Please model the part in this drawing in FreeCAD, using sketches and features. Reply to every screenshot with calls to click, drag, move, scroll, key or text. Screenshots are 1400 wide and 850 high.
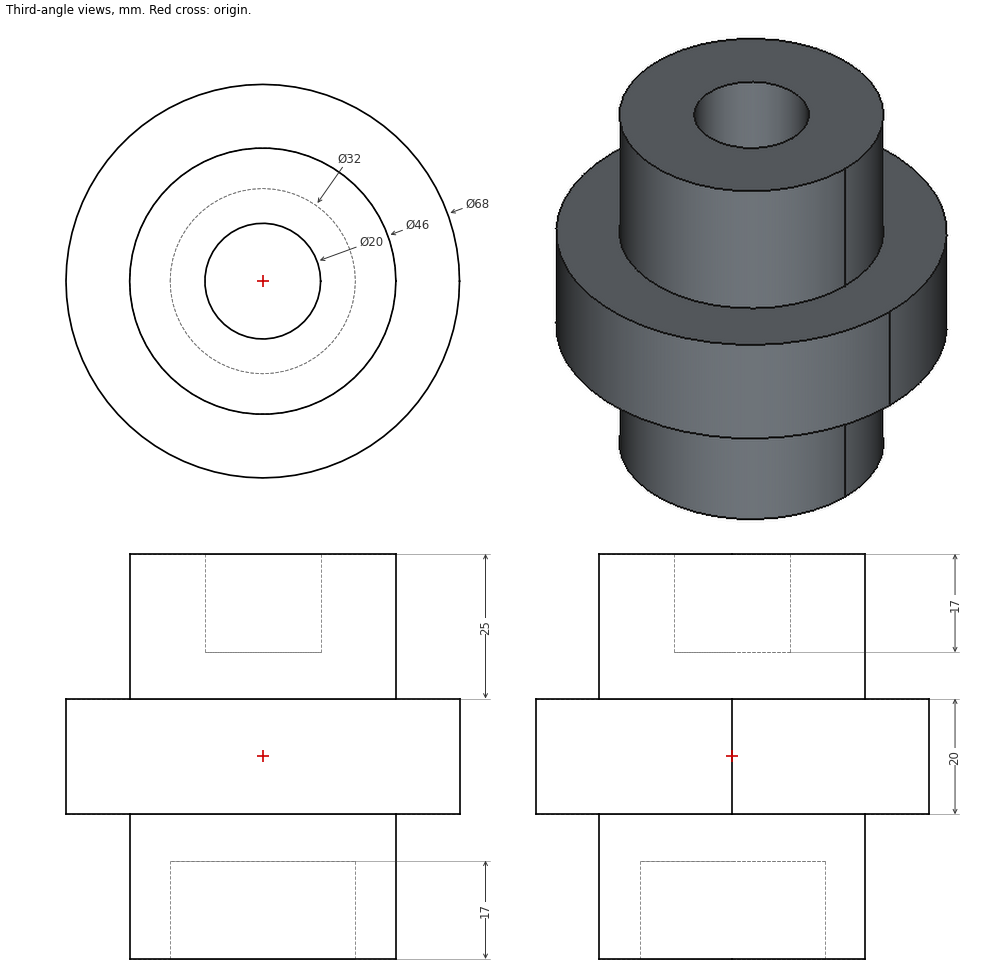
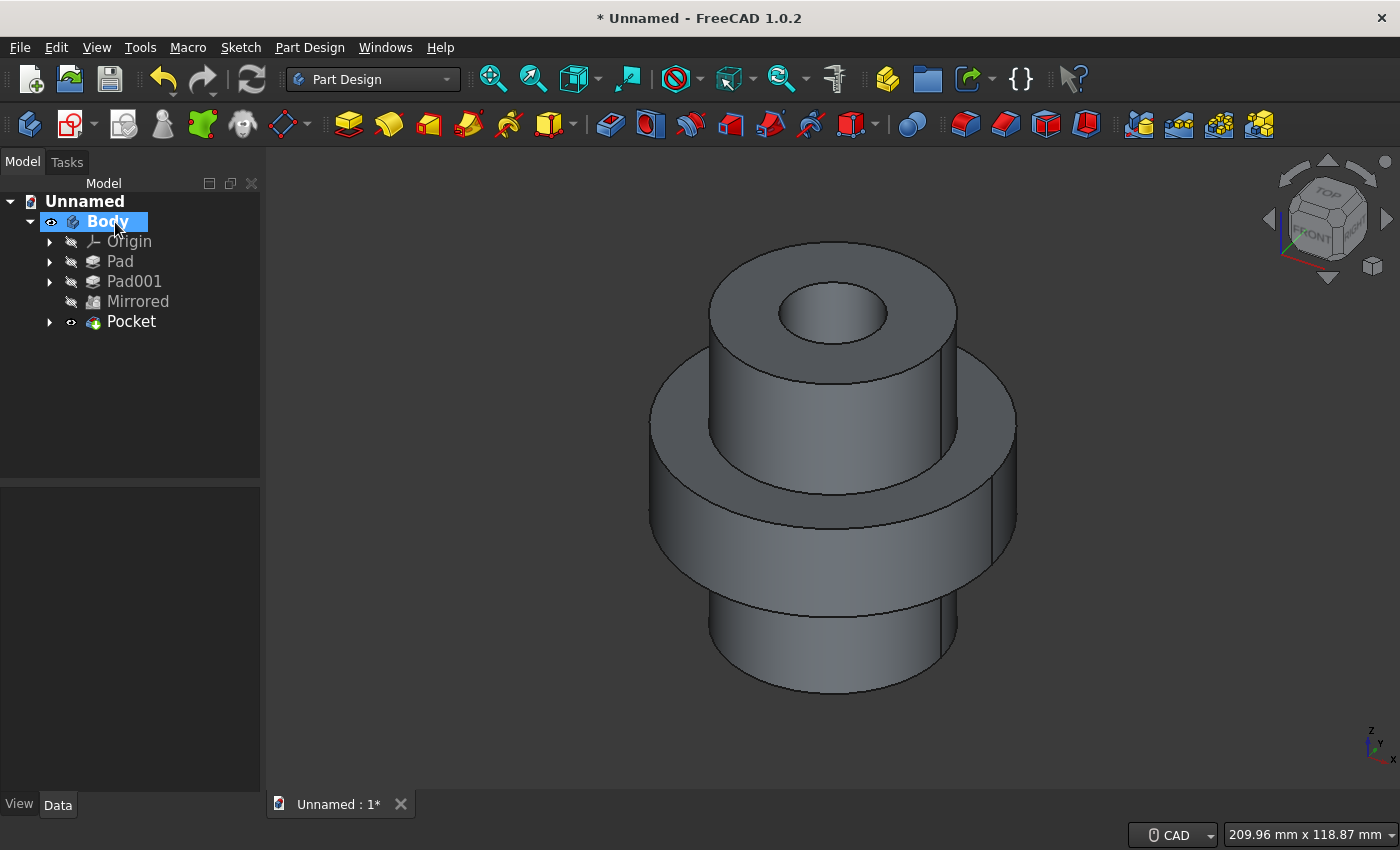
key(5)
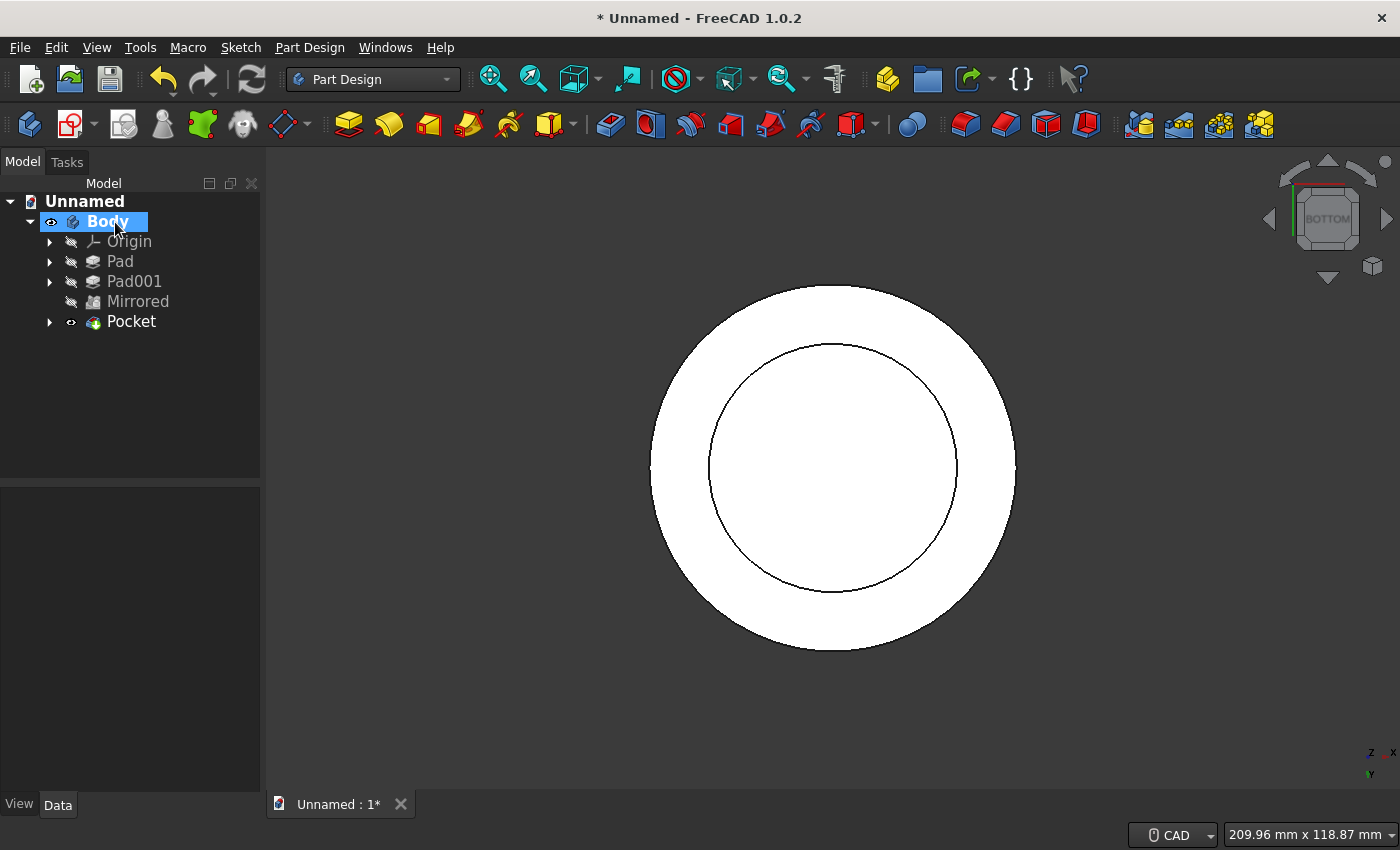
click(833, 467)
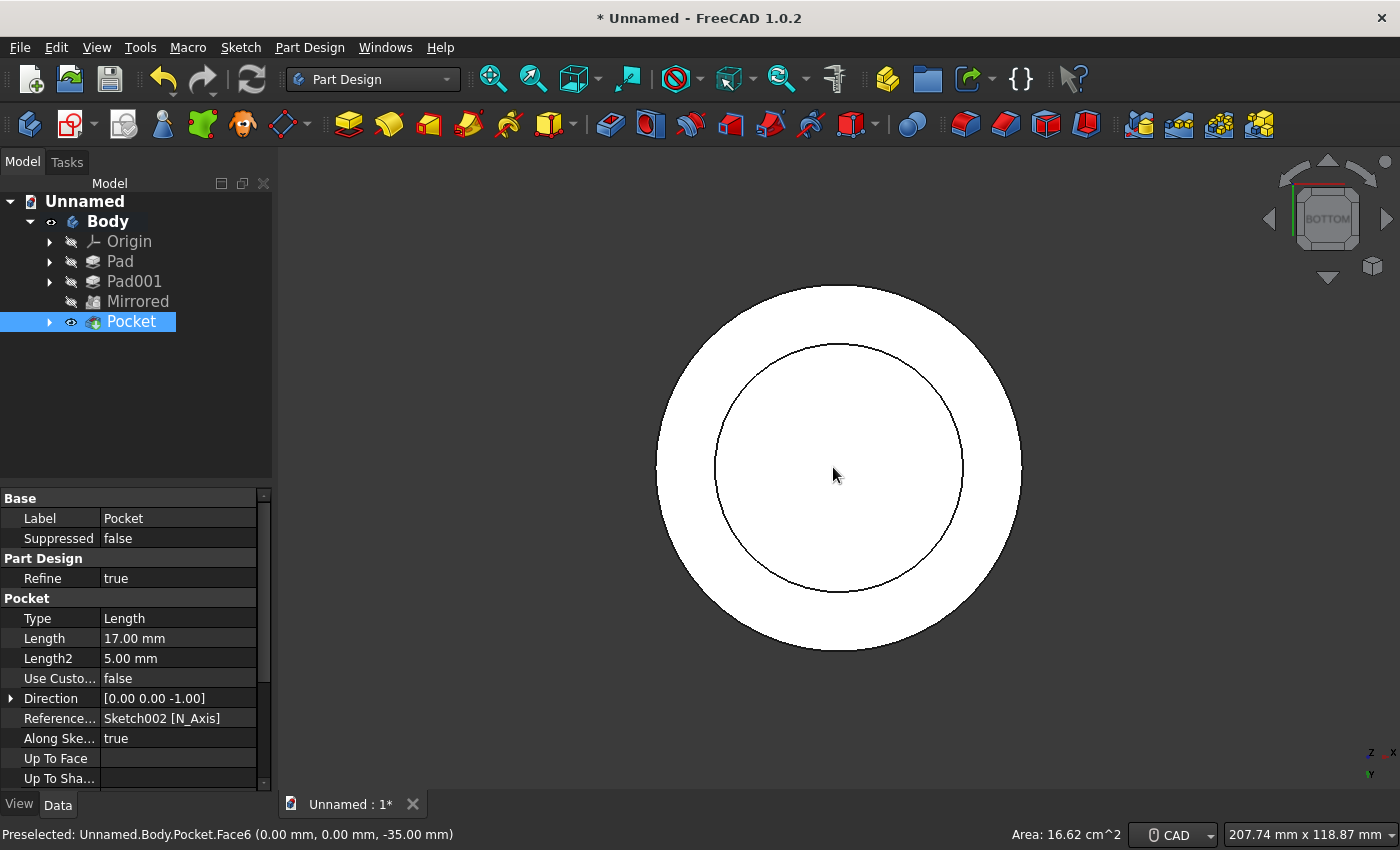
click(70, 124)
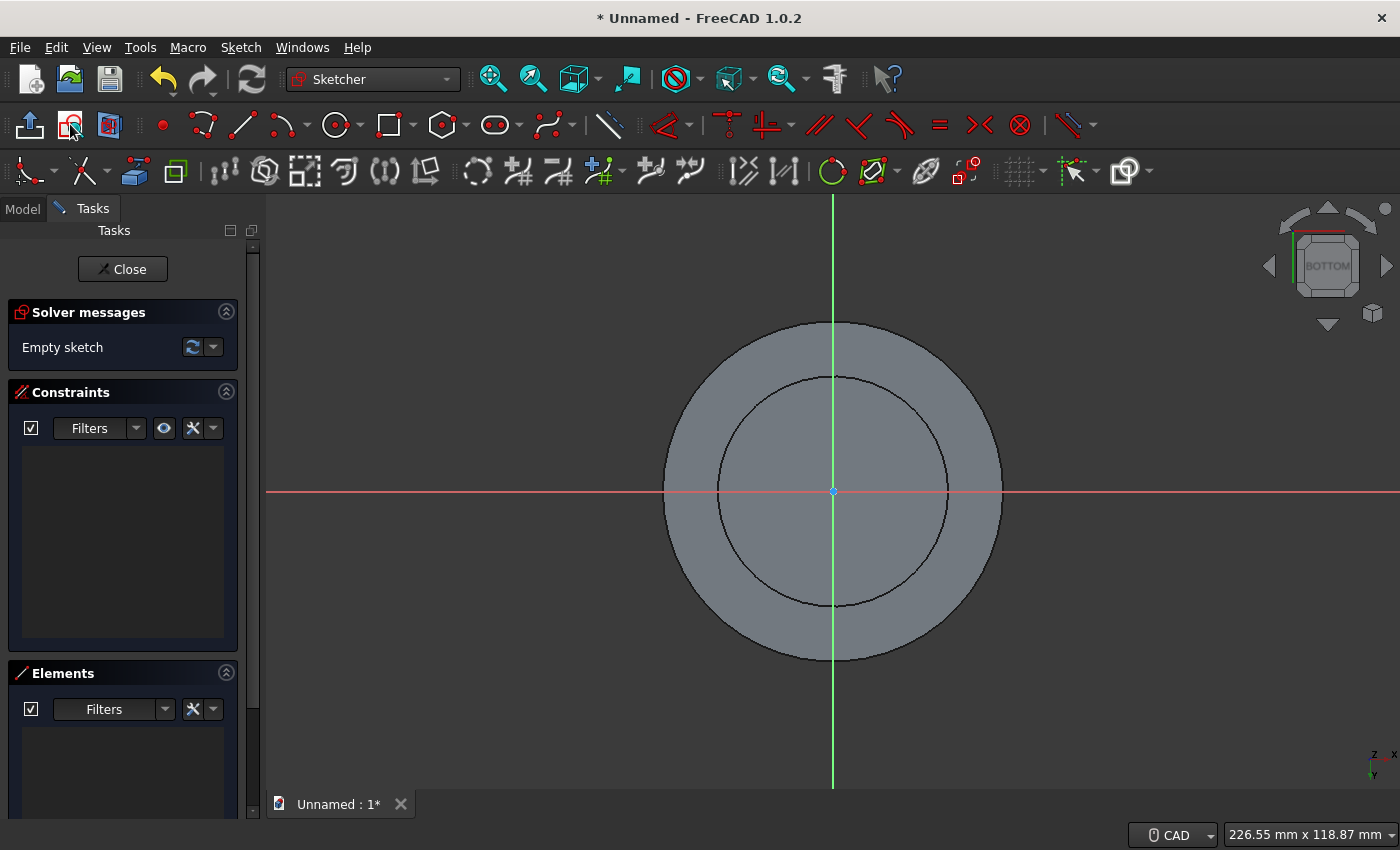
scroll(889, 491, up, 4)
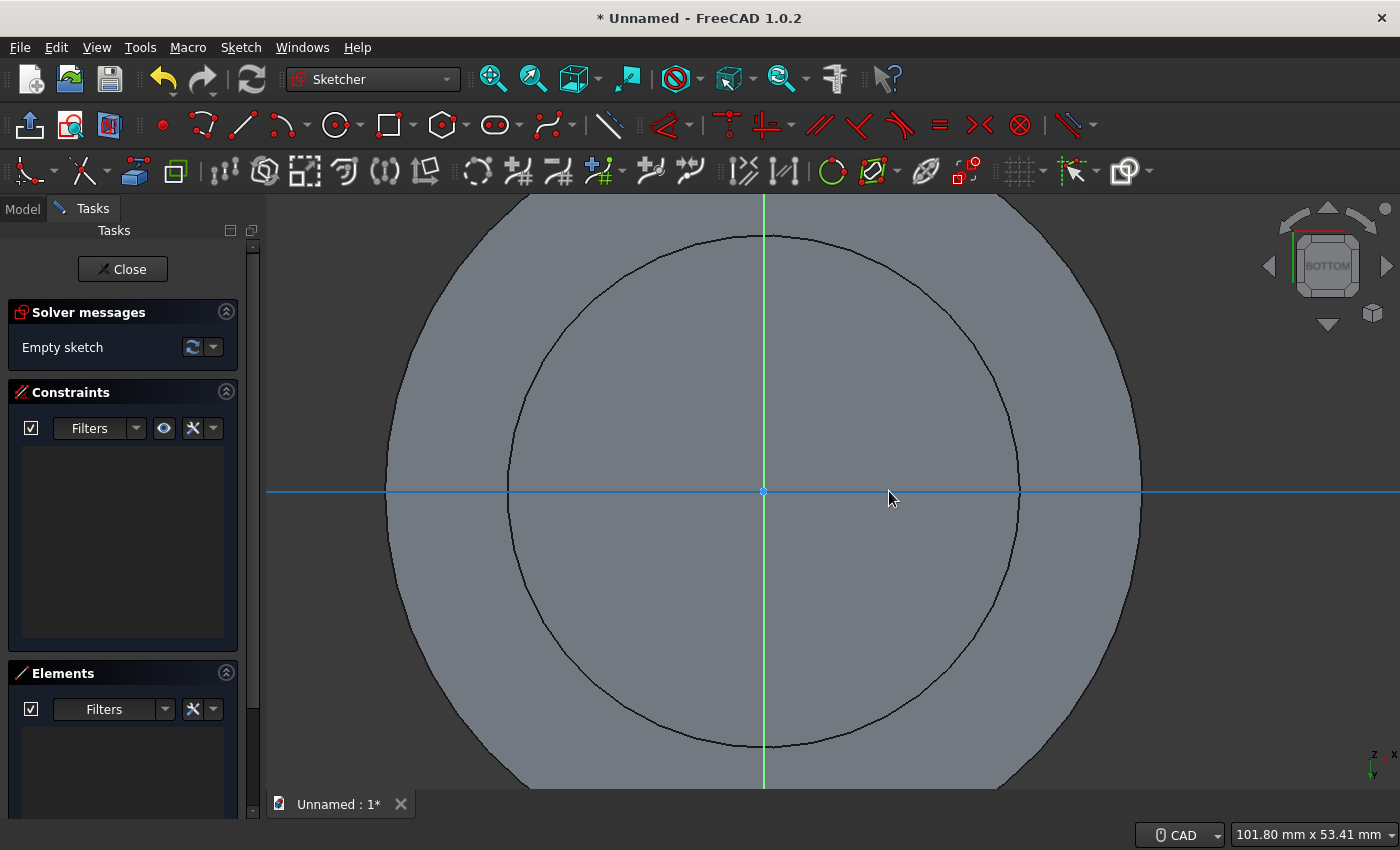
click(336, 126)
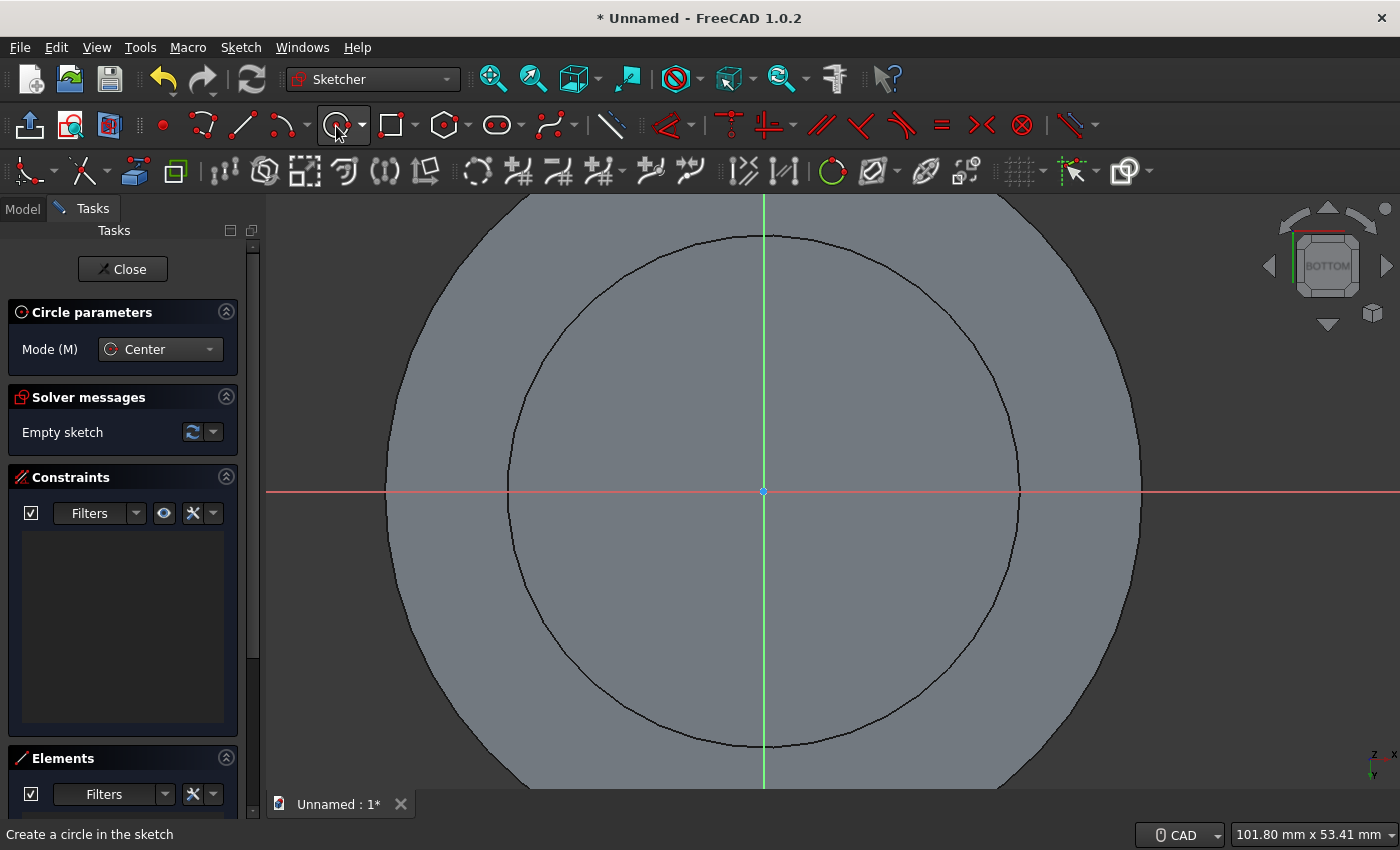
click(764, 492)
move(890, 365)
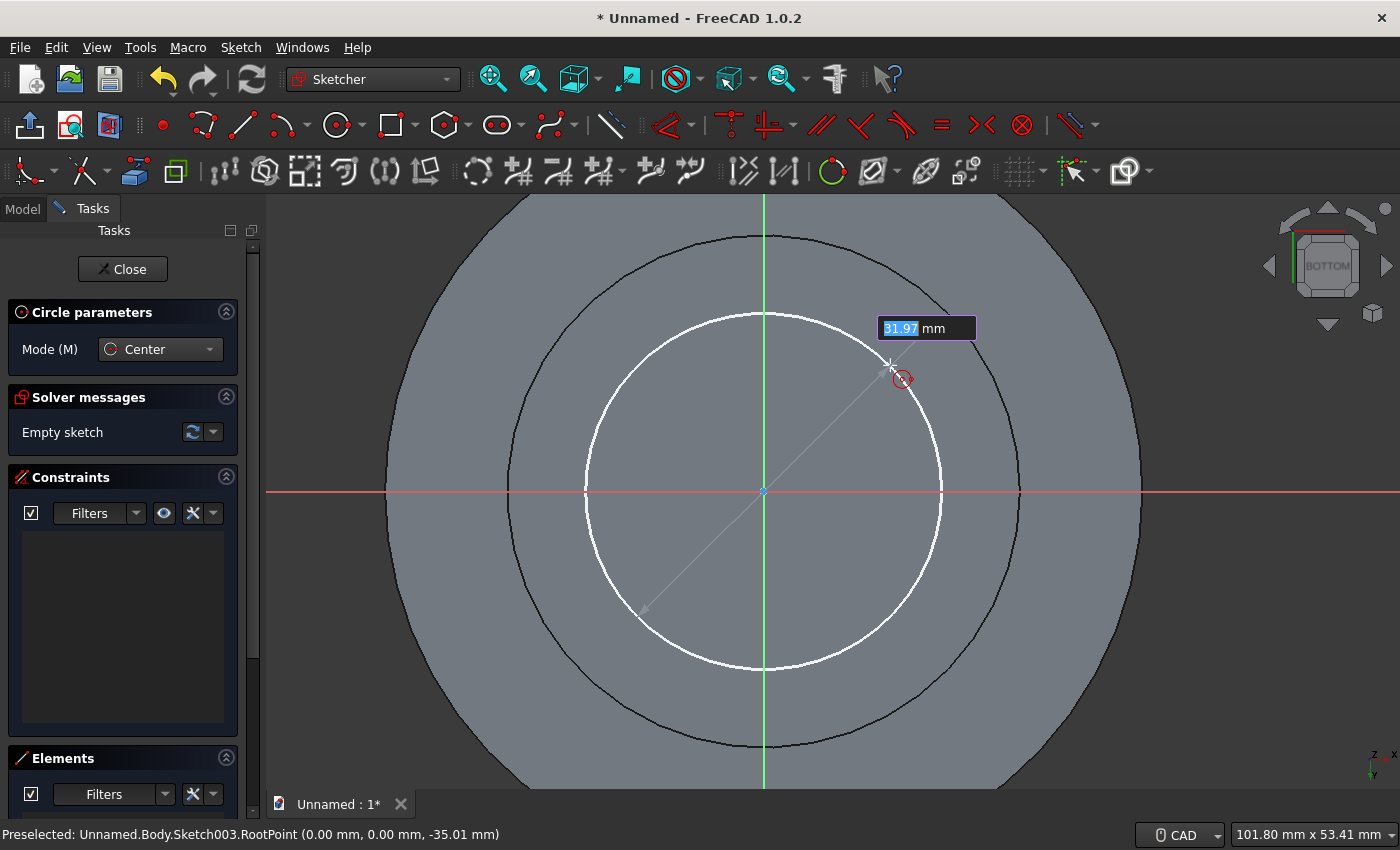
text(32)
key(Return)
key(Escape)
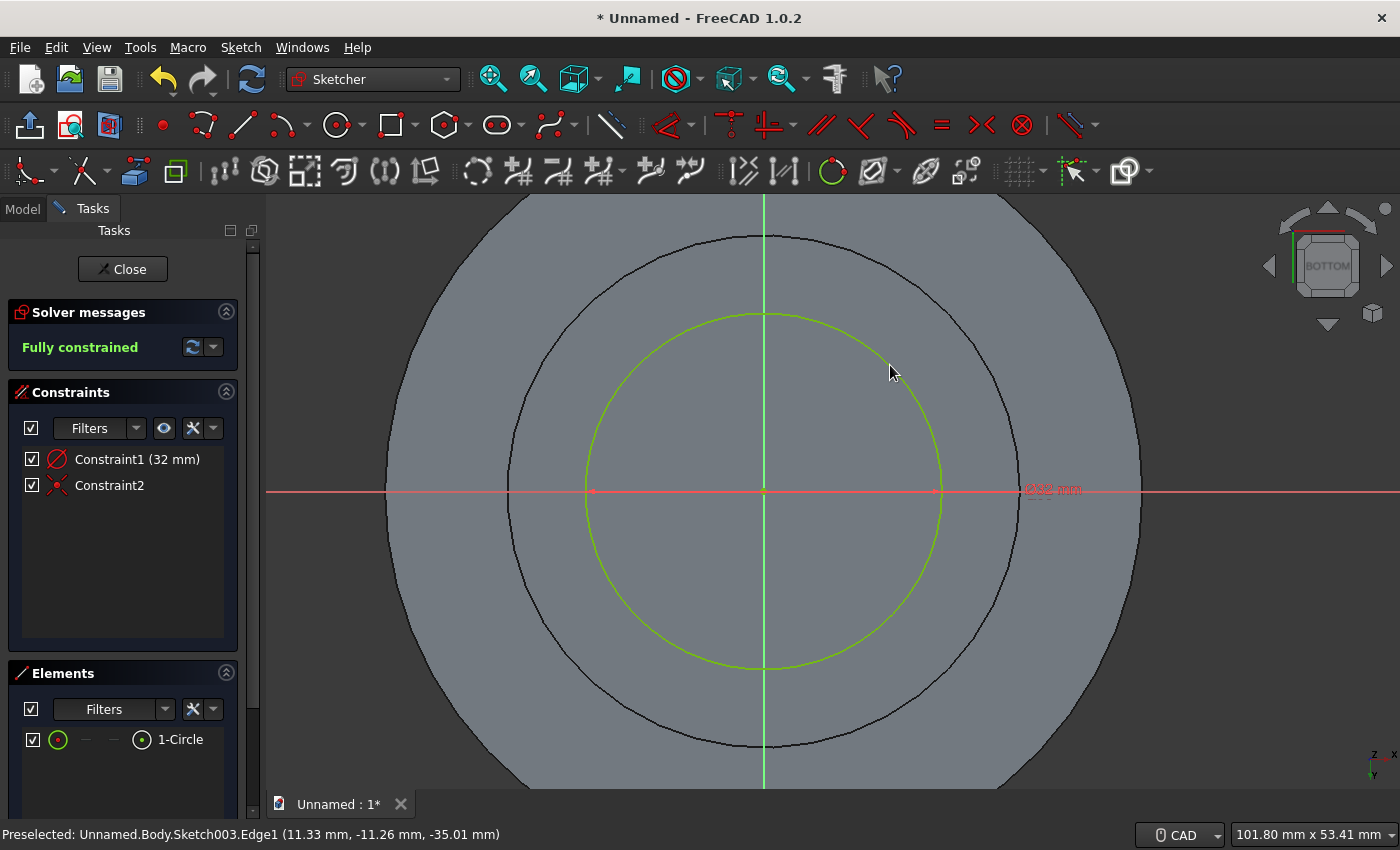
click(123, 269)